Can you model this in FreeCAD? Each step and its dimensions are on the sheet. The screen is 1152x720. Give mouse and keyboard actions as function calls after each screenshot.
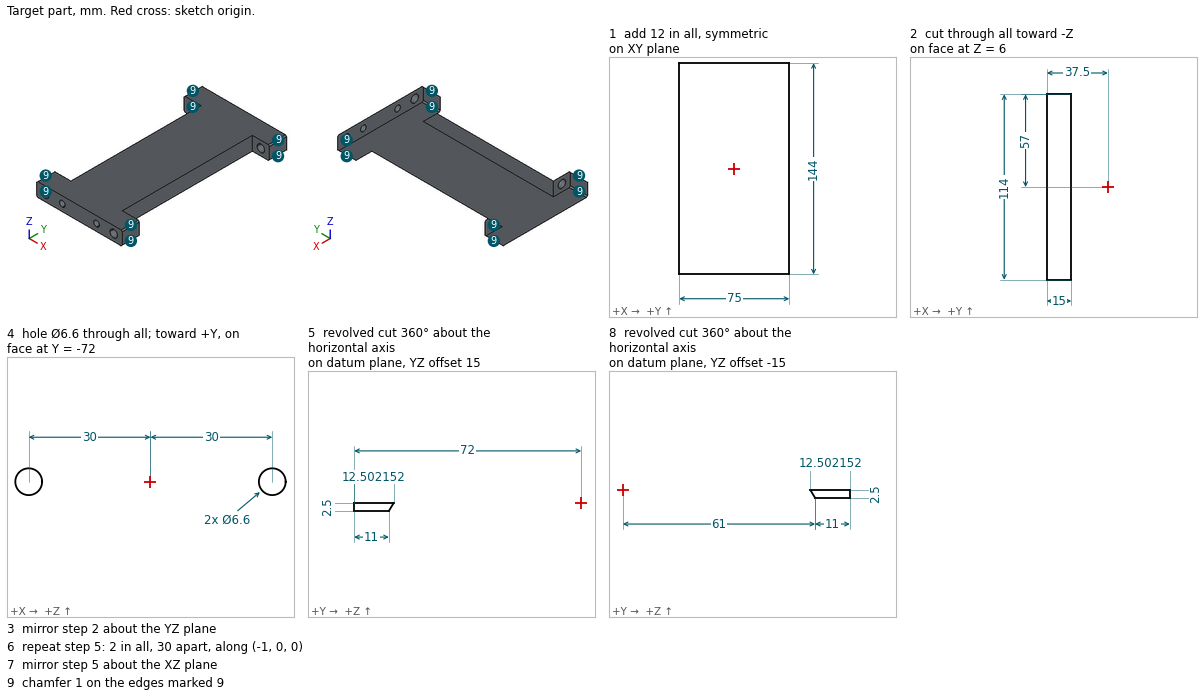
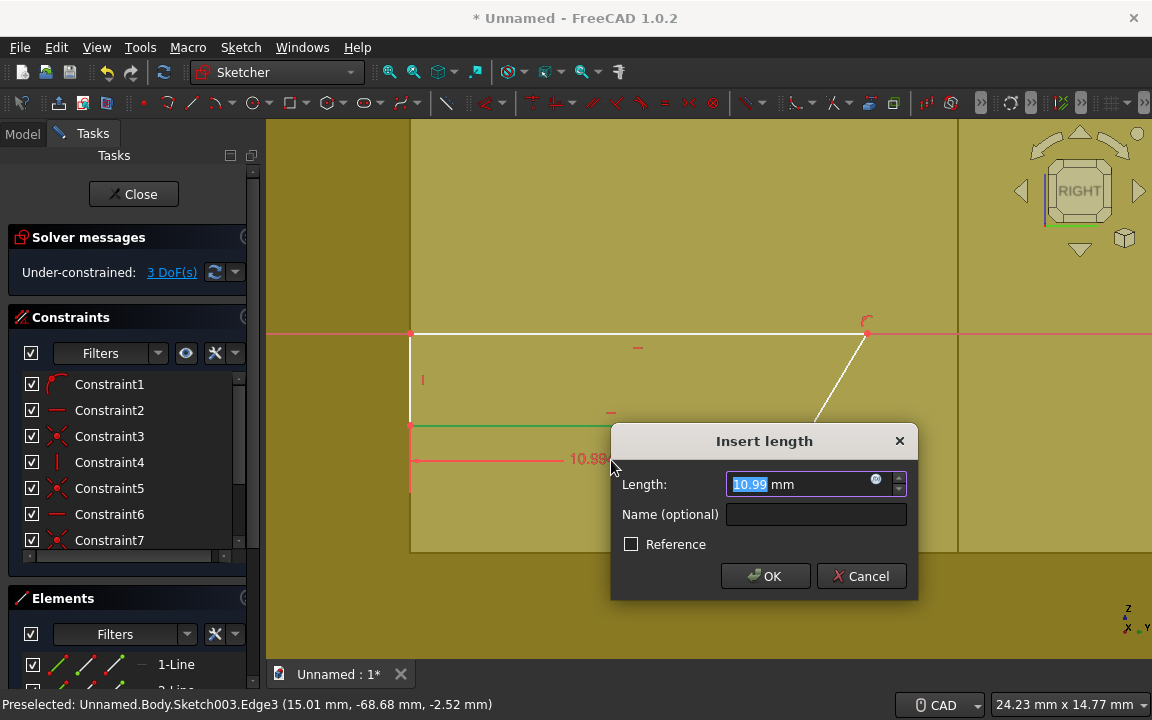
text(11)
key(Return)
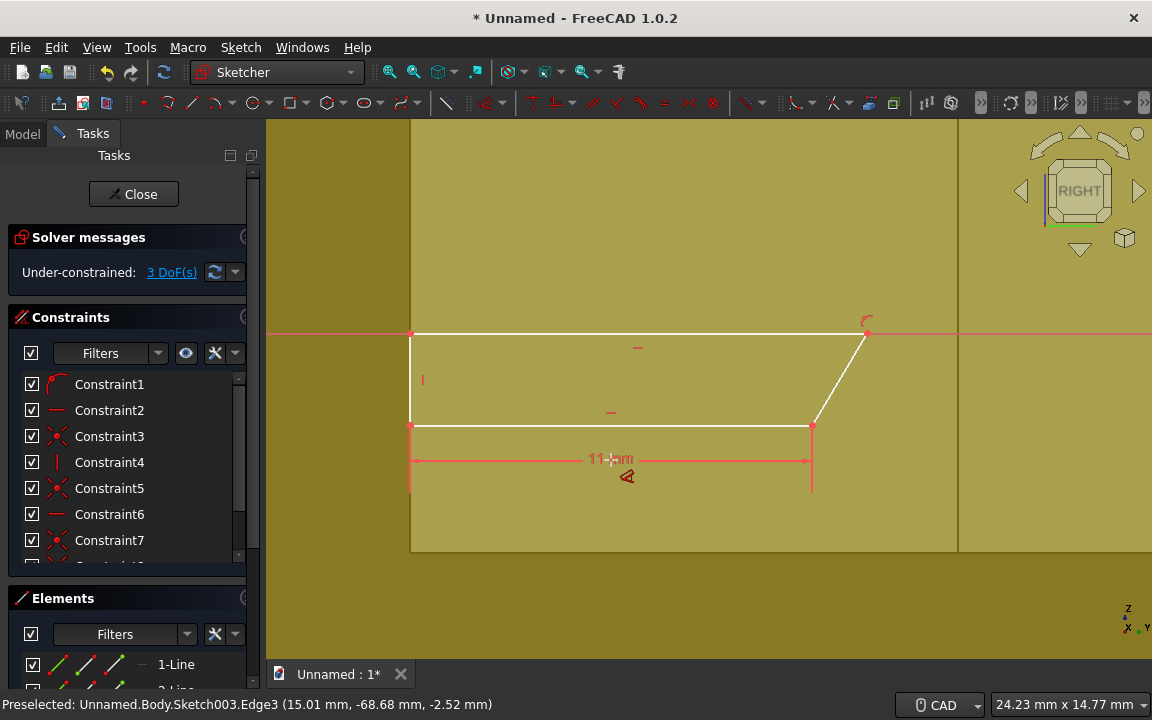
click(410, 361)
click(376, 380)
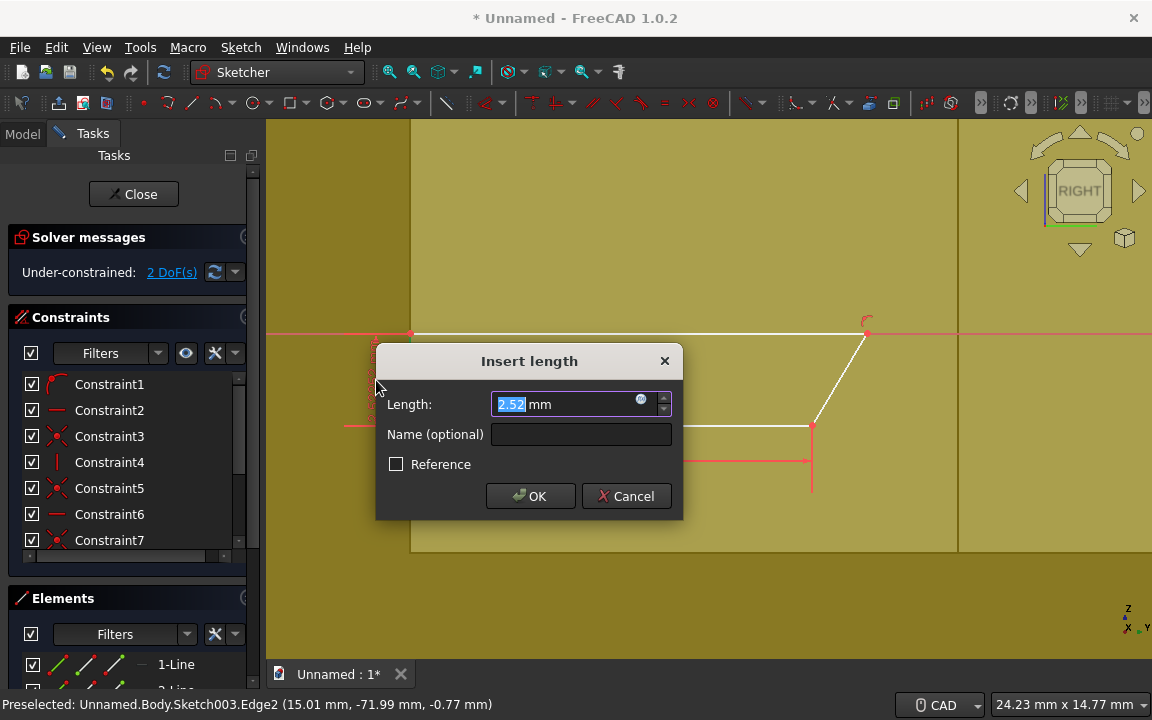
text(2.5)
key(Return)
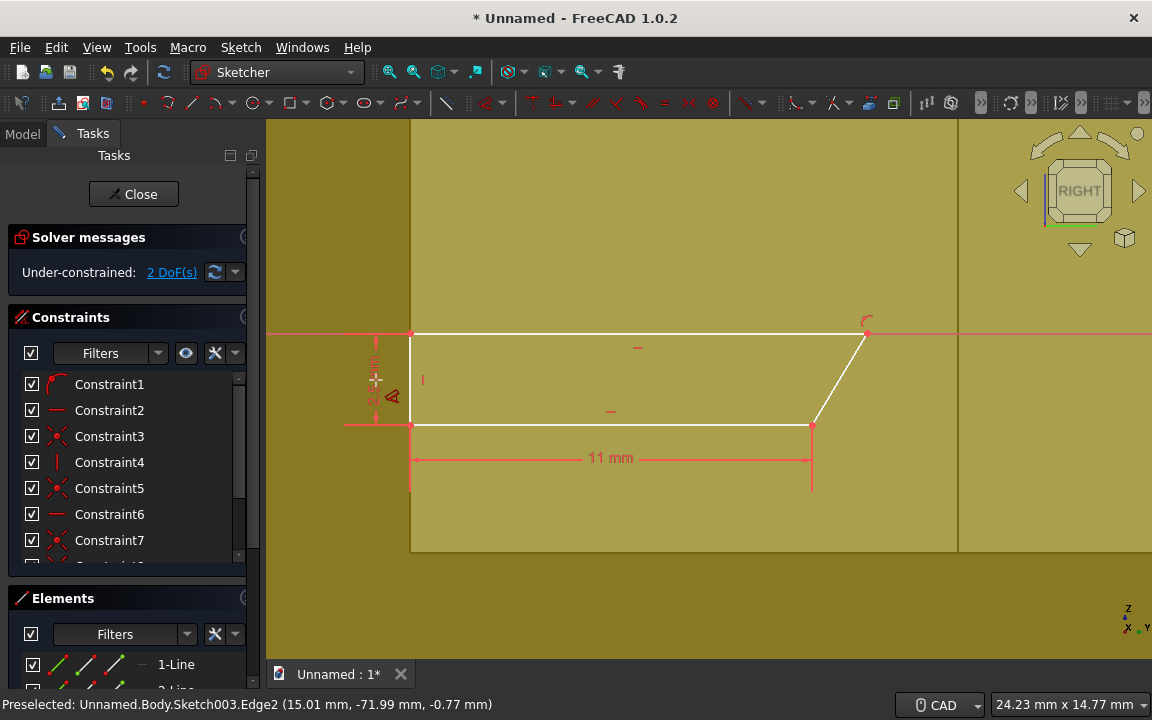
click(410, 334)
click(699, 300)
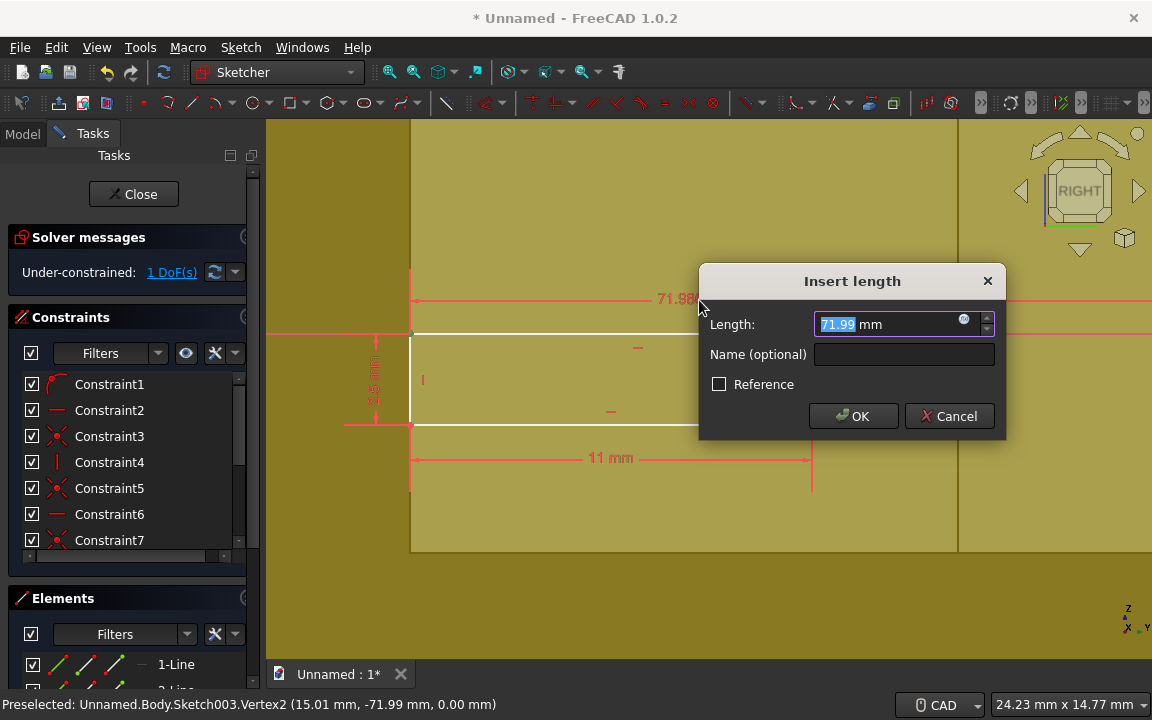
text(72)
key(Return)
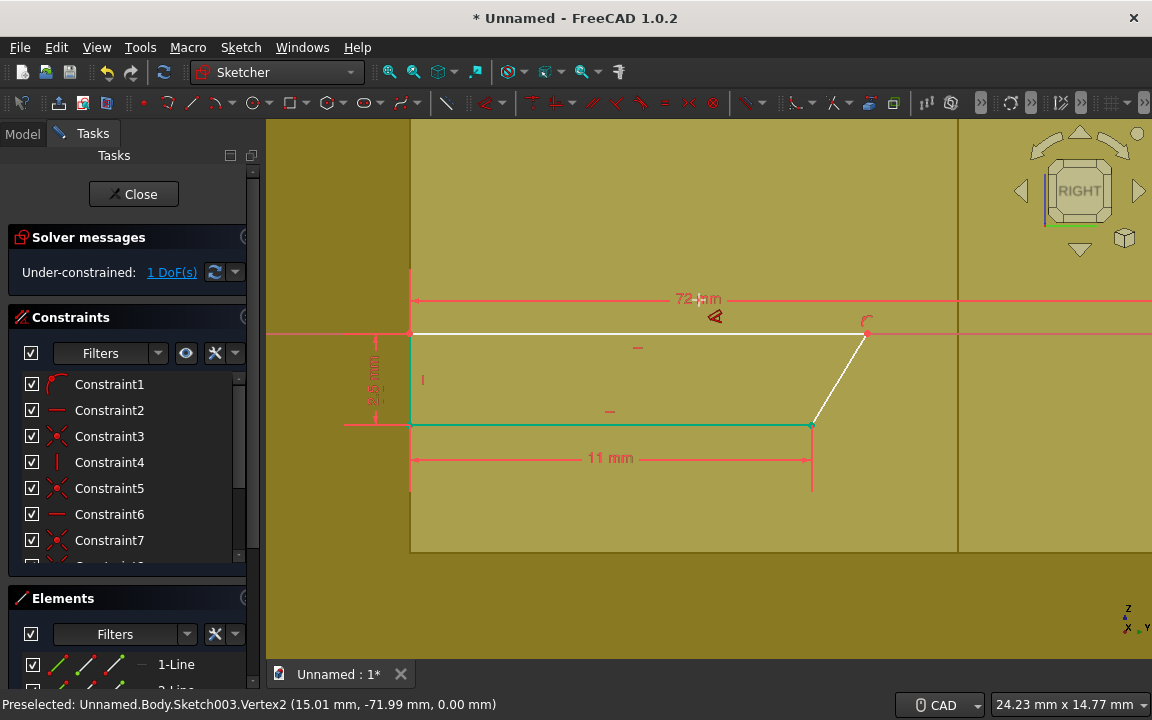
click(730, 334)
click(533, 300)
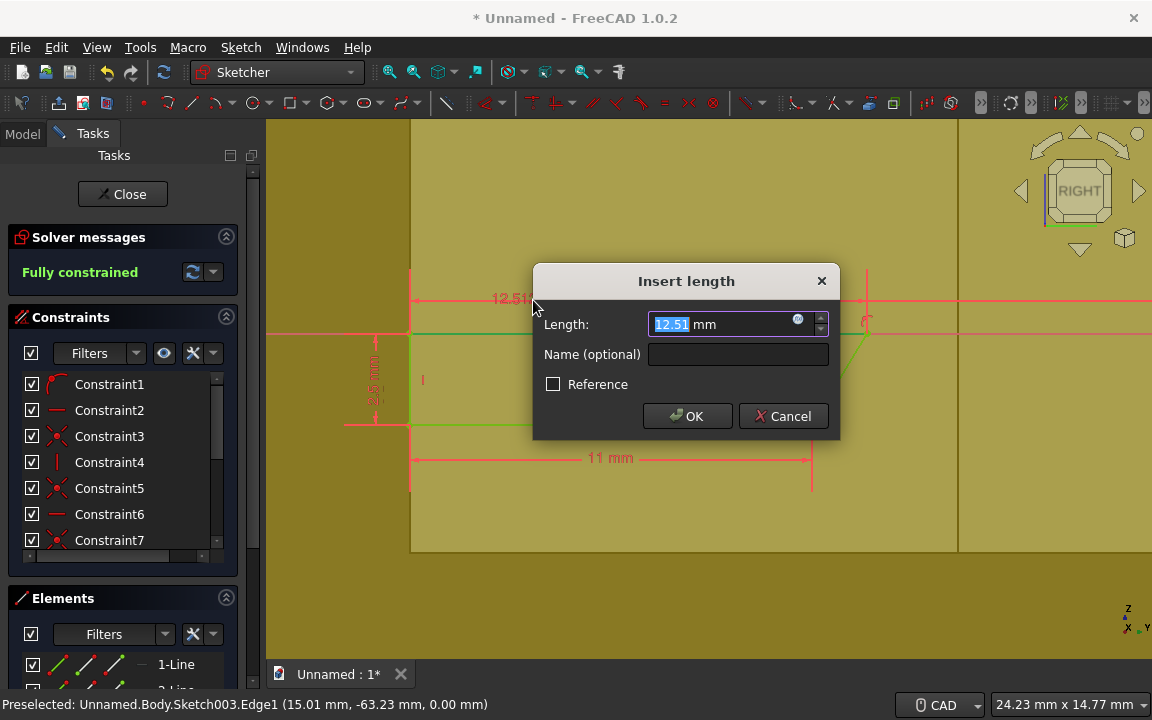
text(12.502152)
key(Return)
key(Escape)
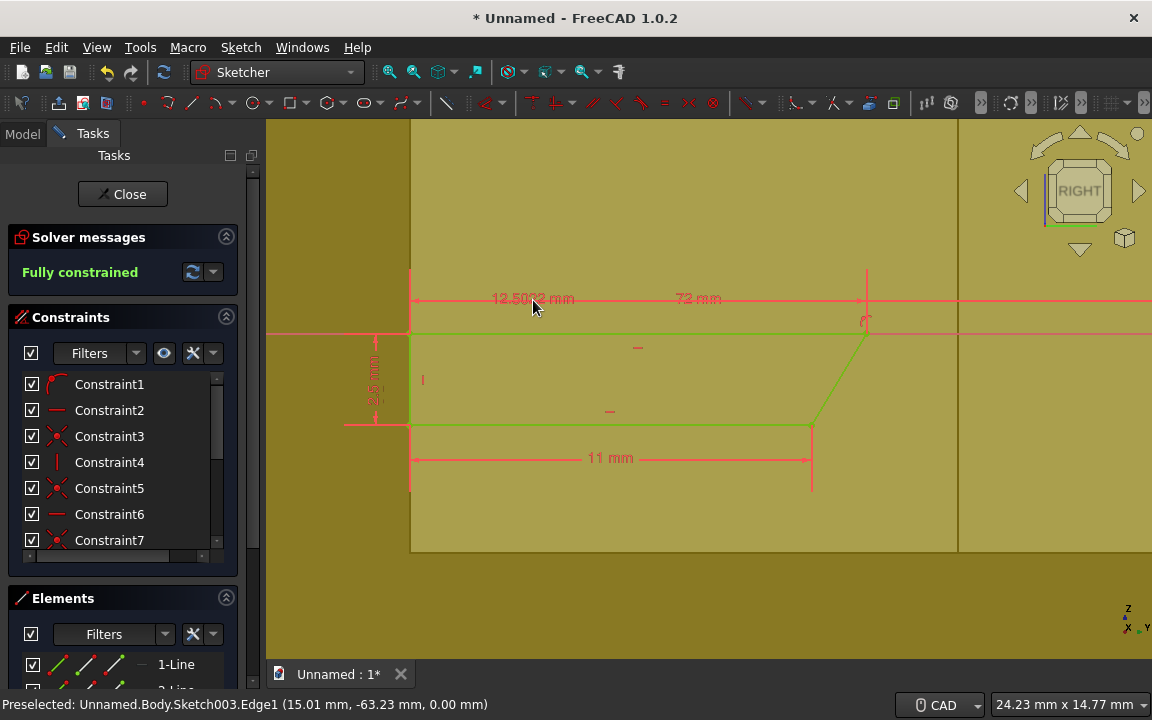
click(123, 194)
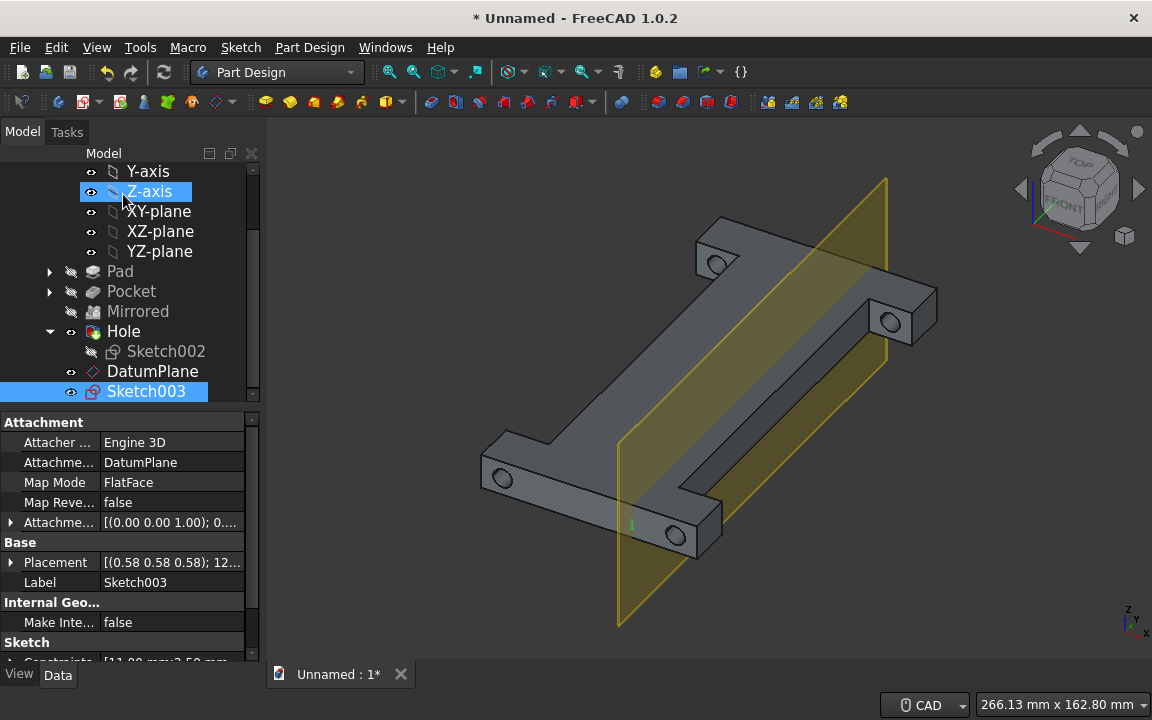
click(480, 102)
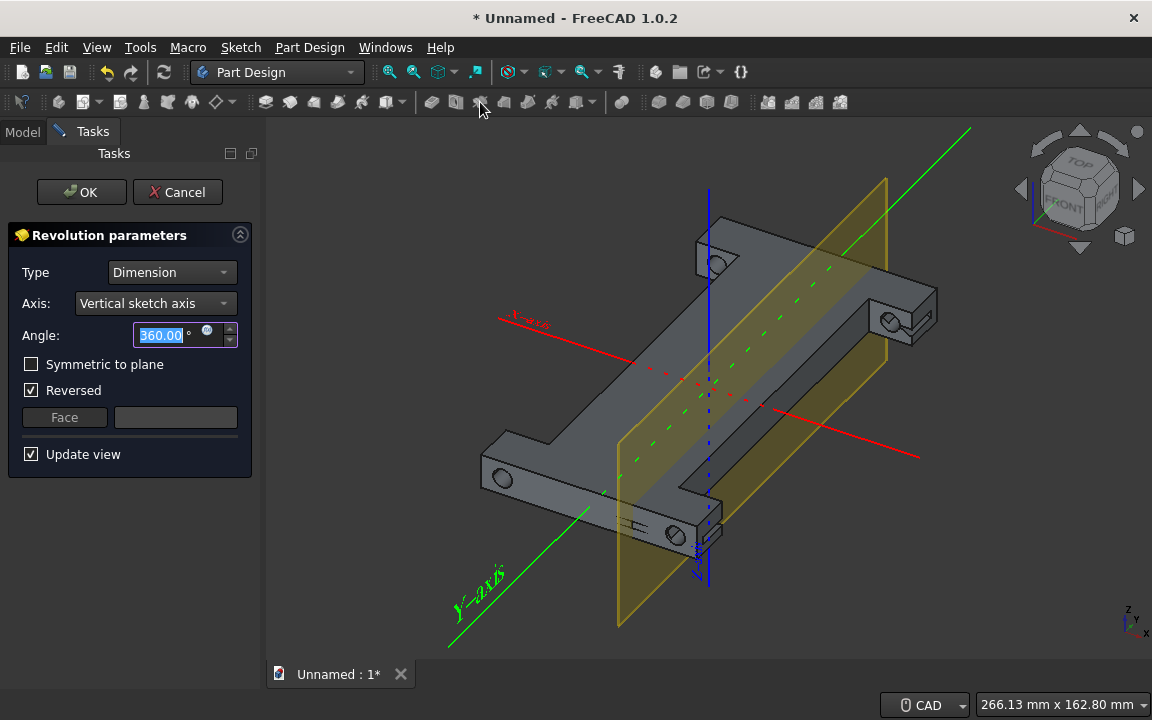
click(156, 304)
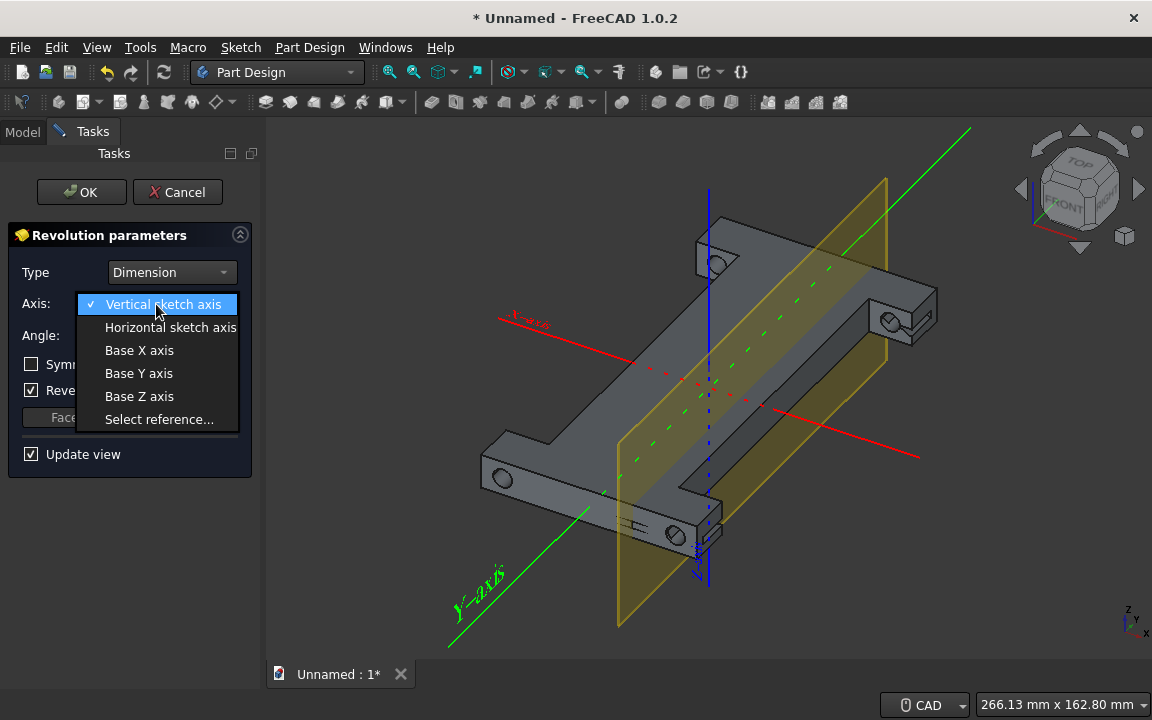
click(156, 328)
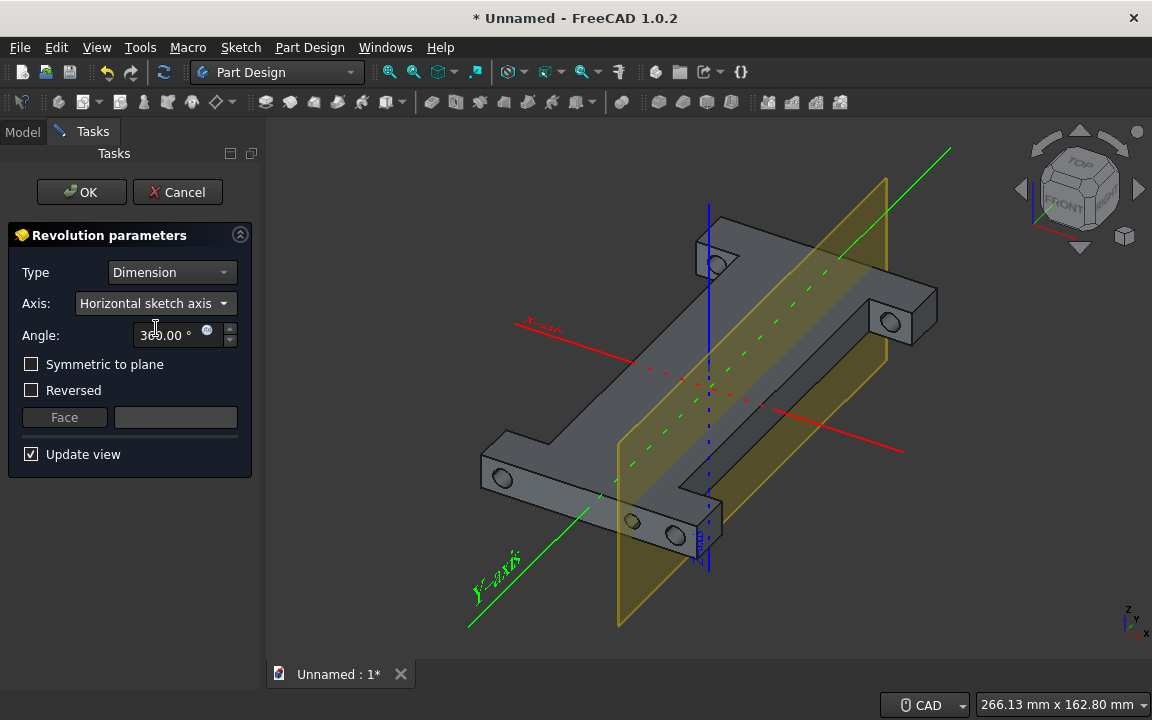
click(82, 192)